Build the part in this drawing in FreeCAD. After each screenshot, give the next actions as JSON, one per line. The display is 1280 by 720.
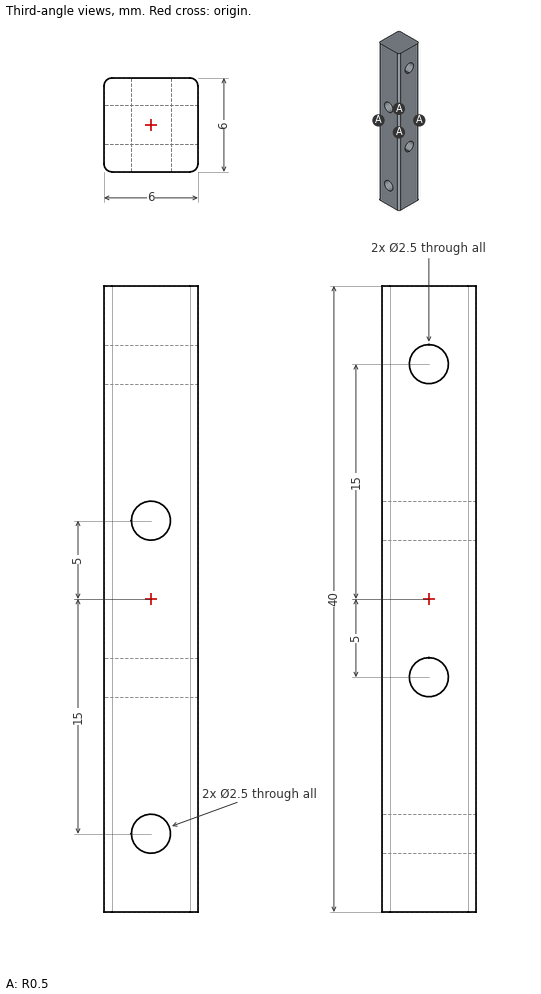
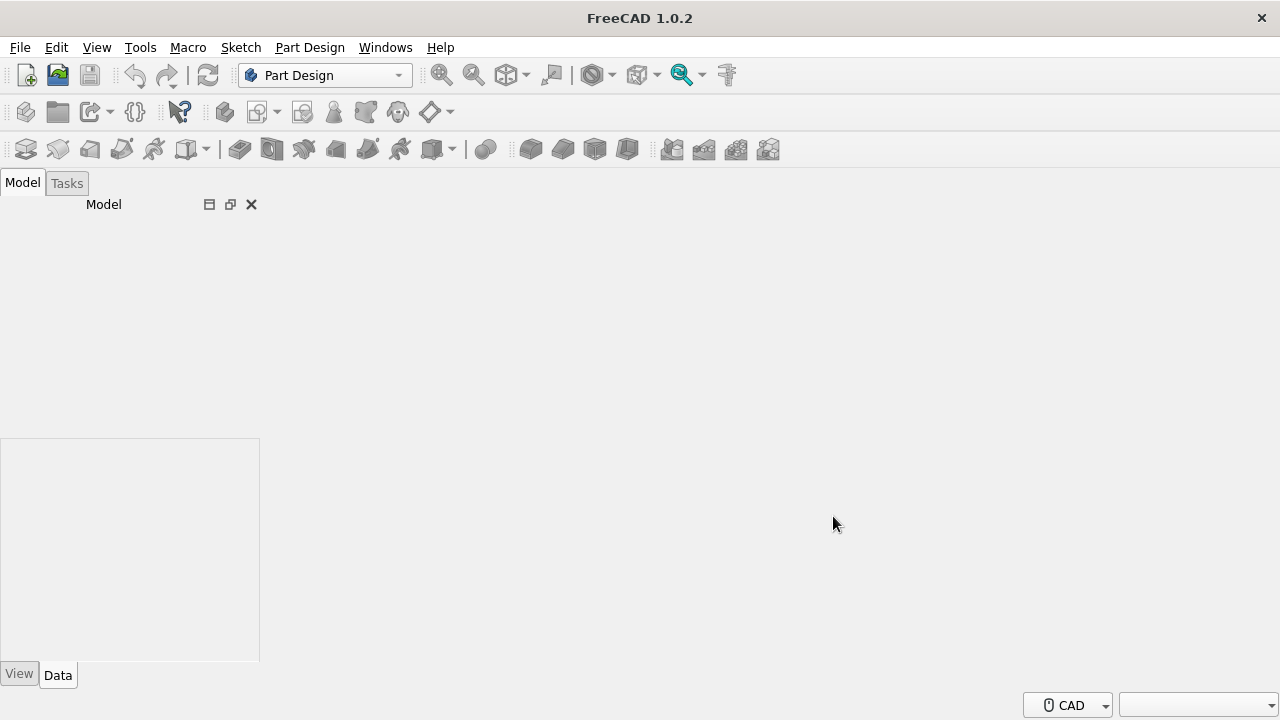
{"action": "left_click", "coordinate": [26, 76]}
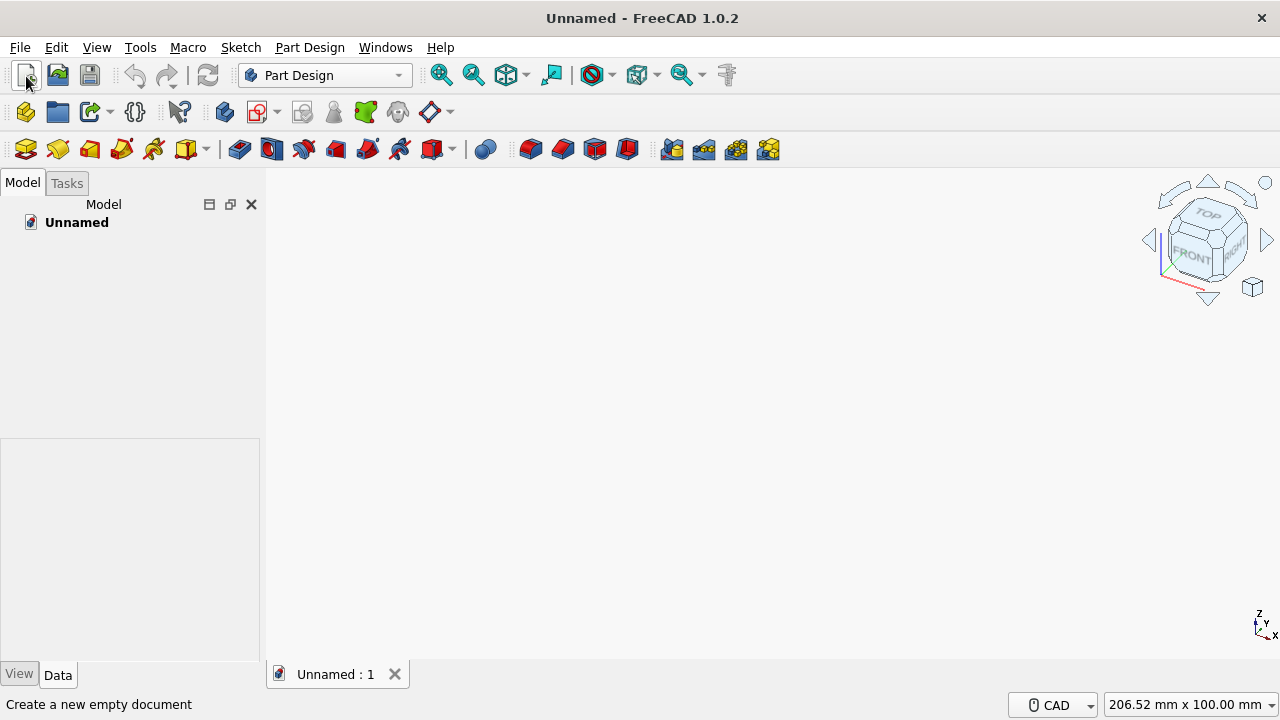
{"action": "left_click", "coordinate": [258, 112]}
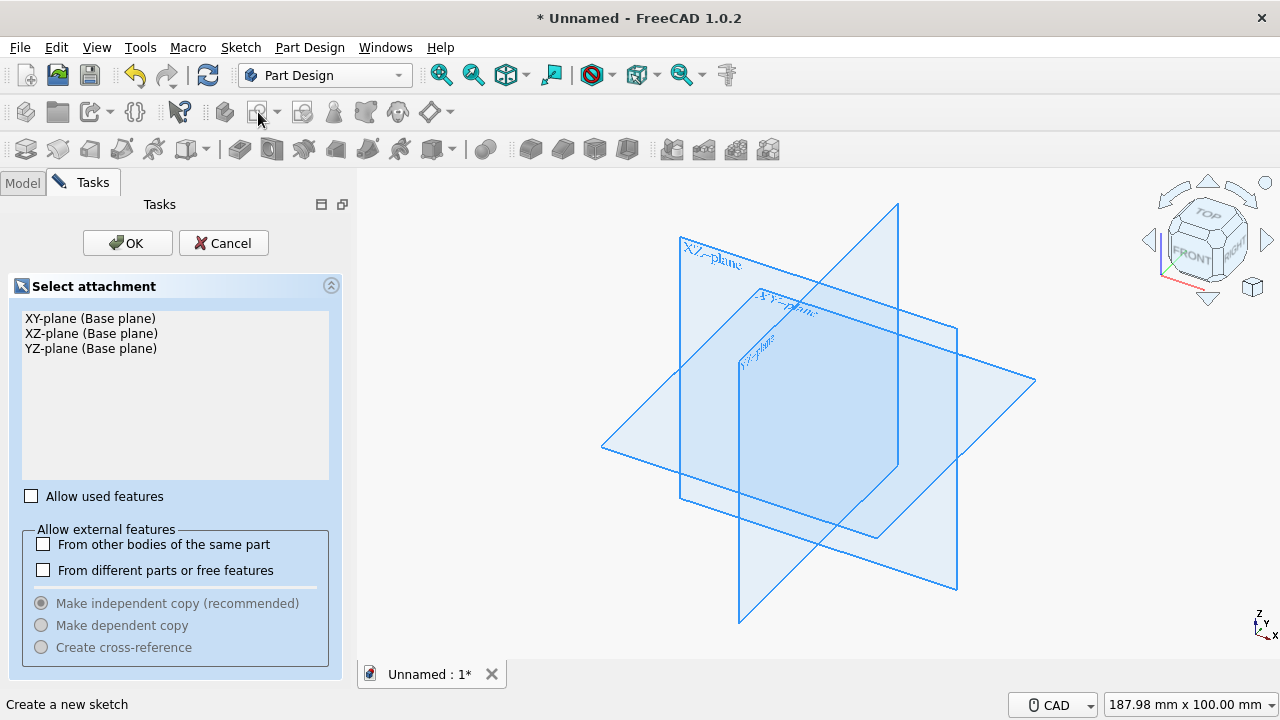
{"action": "left_click", "coordinate": [82, 318]}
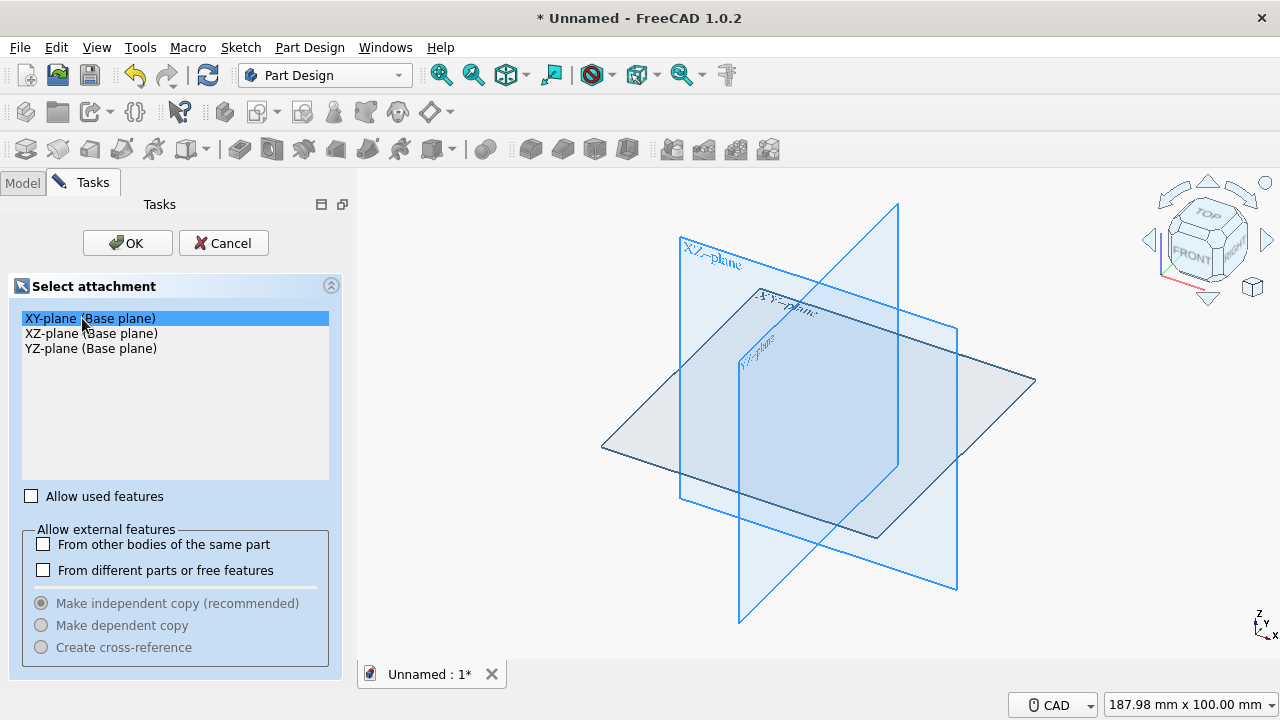
{"action": "left_click", "coordinate": [128, 243]}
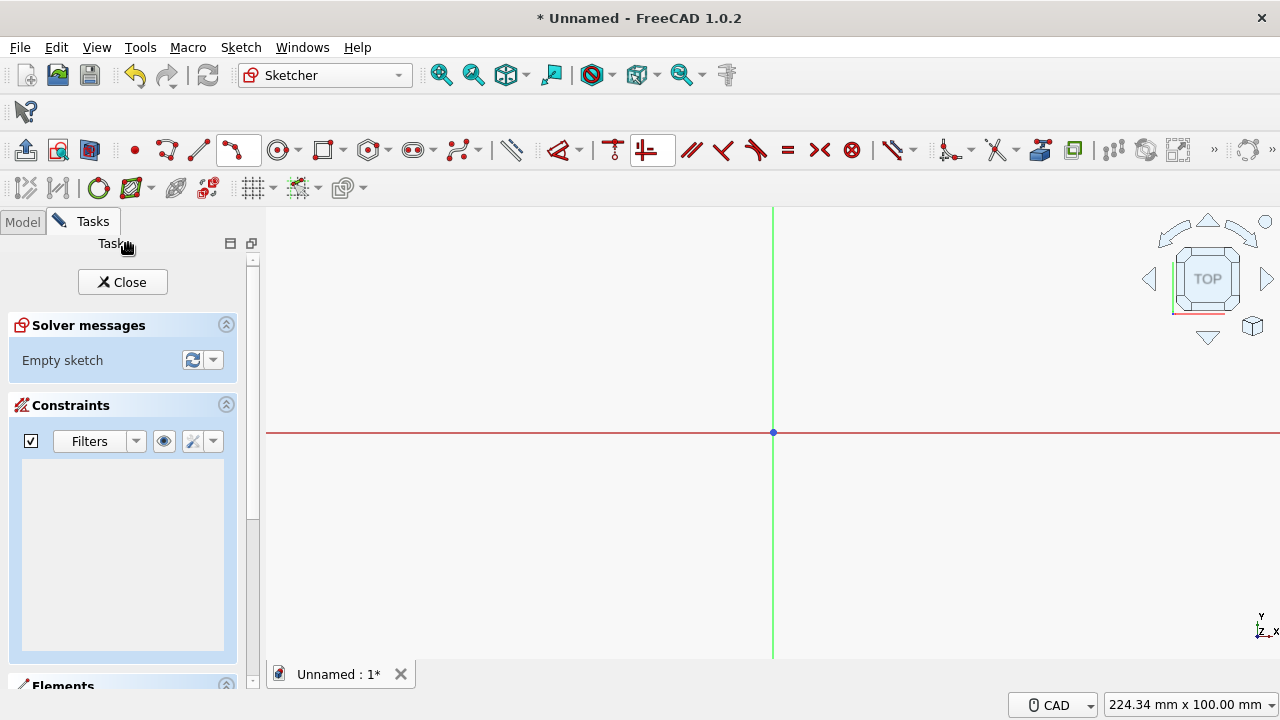
{"action": "scroll", "coordinate": [780, 433], "scroll_direction": "up", "scroll_amount": 12}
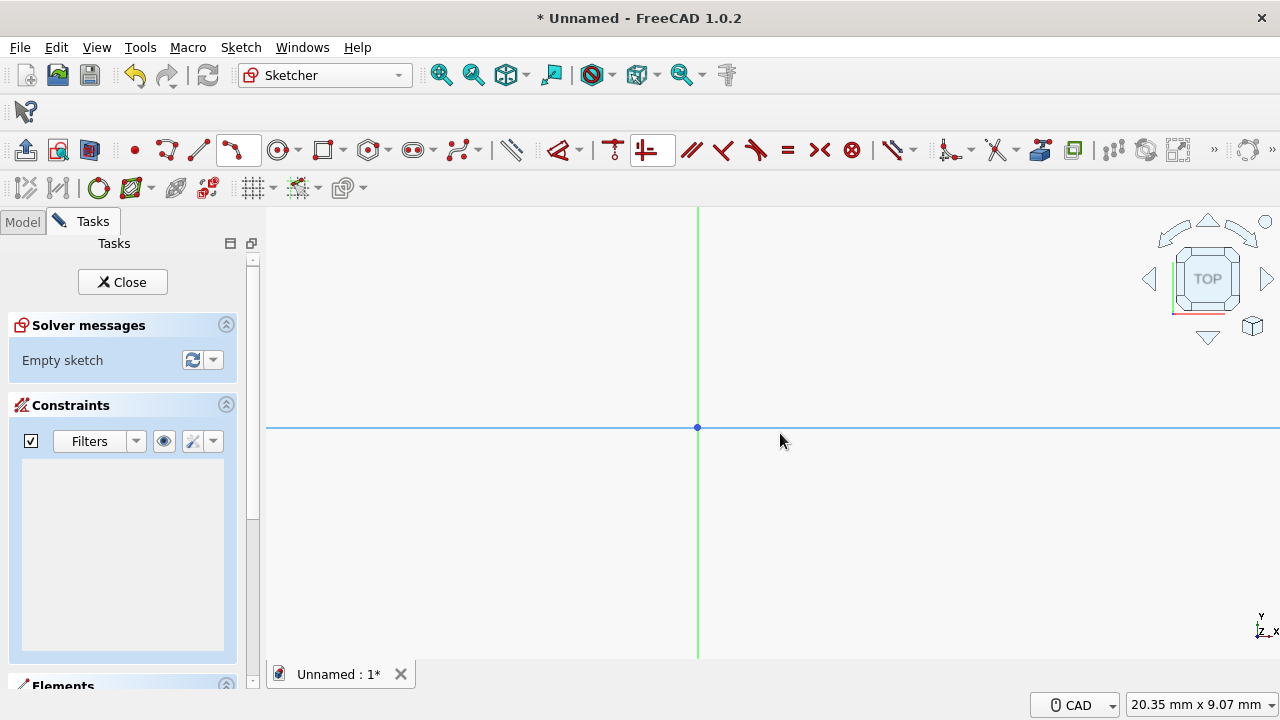
{"action": "left_click", "coordinate": [346, 150]}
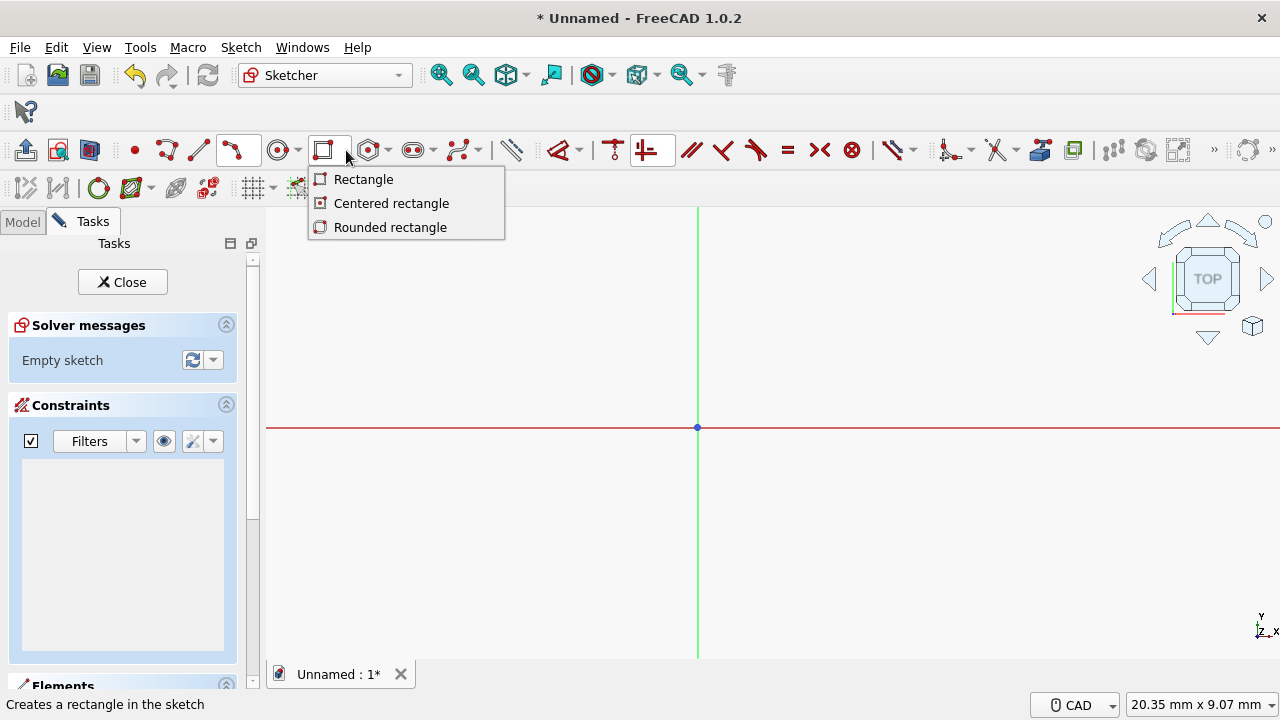
{"action": "left_click", "coordinate": [406, 203]}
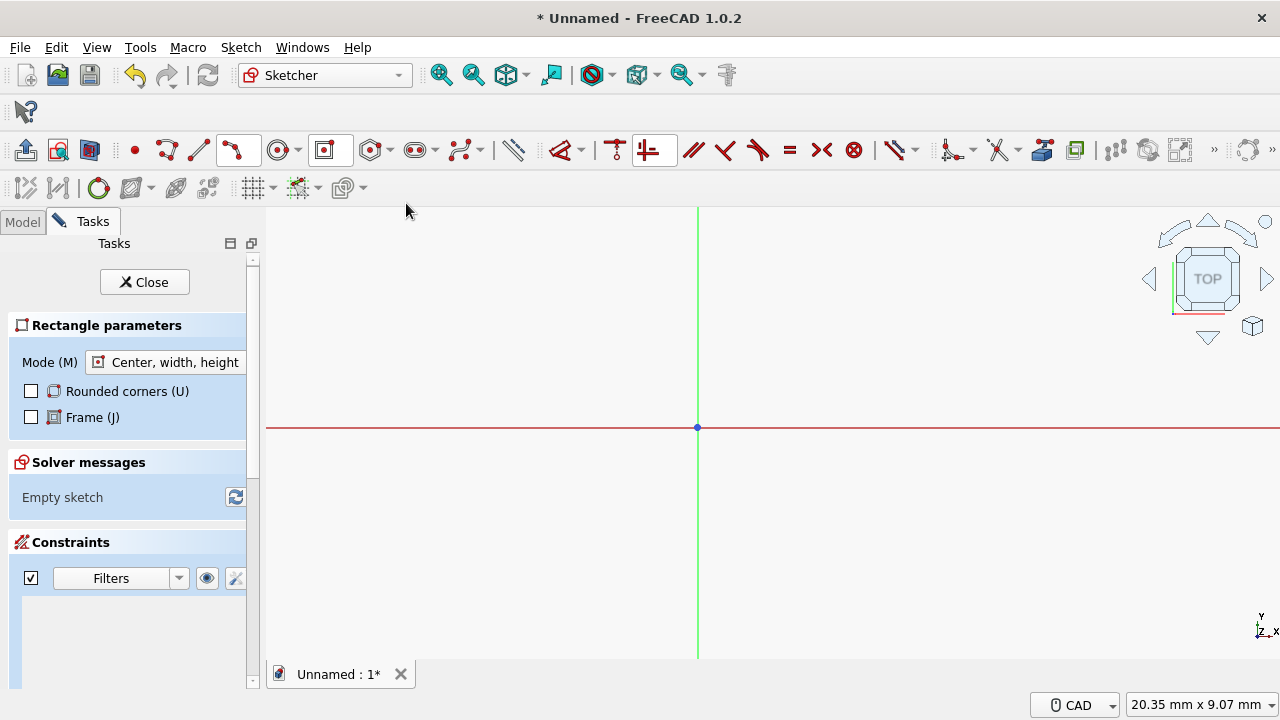
{"action": "left_click", "coordinate": [698, 428]}
{"action": "left_click", "coordinate": [847, 279]}
{"action": "key", "text": "Escape"}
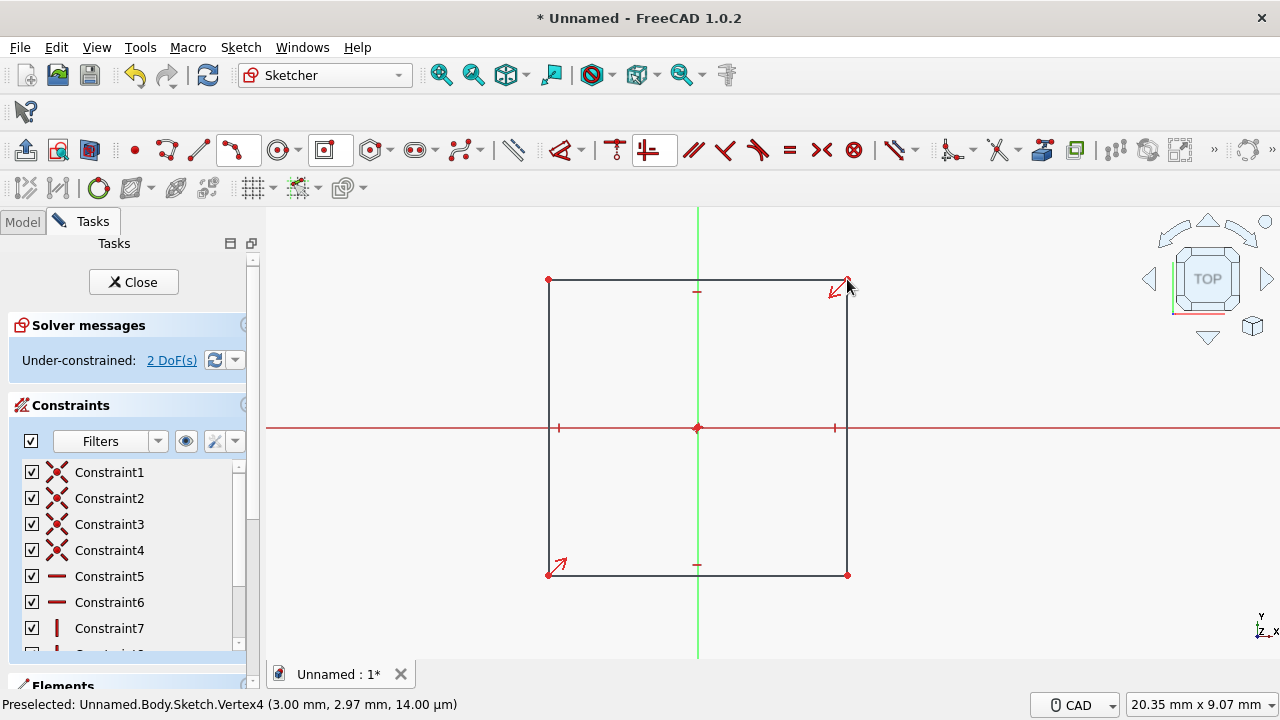
{"action": "left_click", "coordinate": [560, 150]}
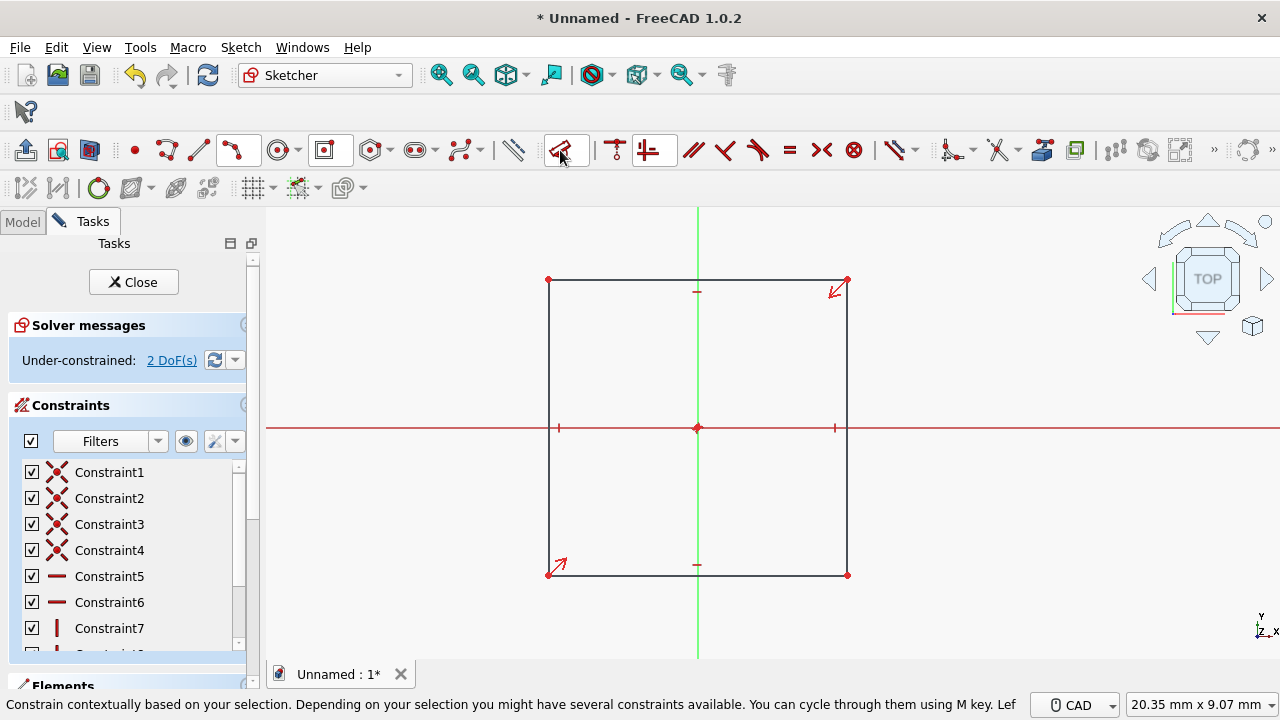
{"action": "left_click", "coordinate": [638, 576]}
{"action": "left_click", "coordinate": [629, 610]}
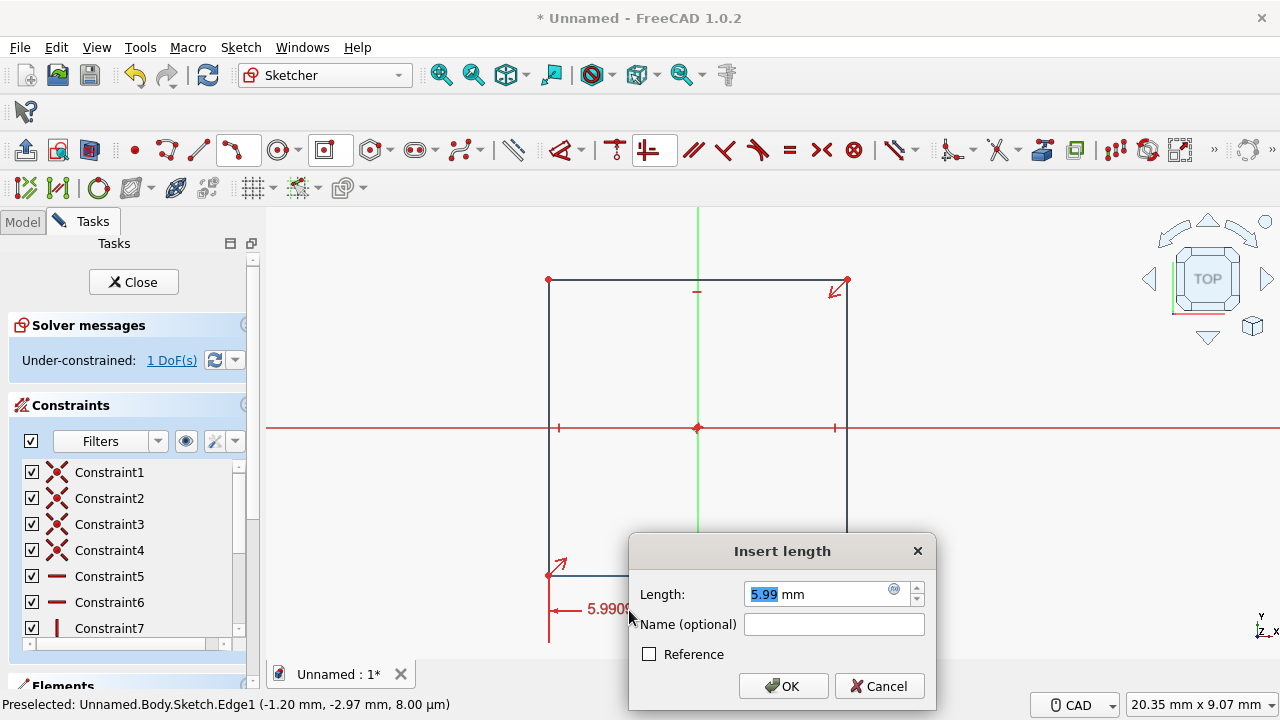
{"action": "type", "text": "6"}
{"action": "key", "text": "Return"}